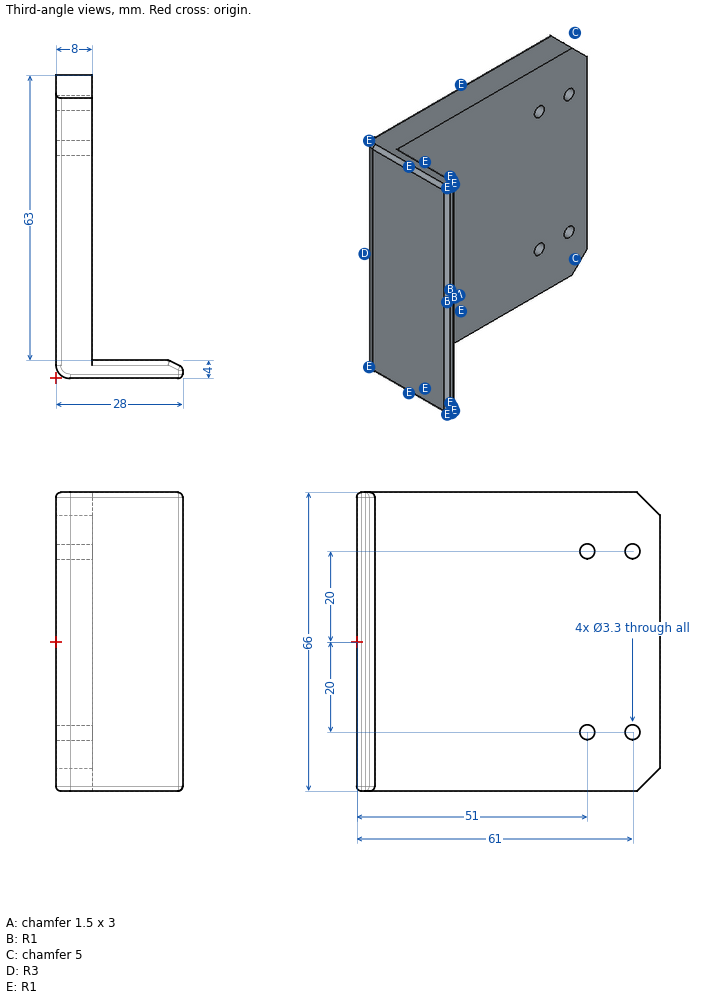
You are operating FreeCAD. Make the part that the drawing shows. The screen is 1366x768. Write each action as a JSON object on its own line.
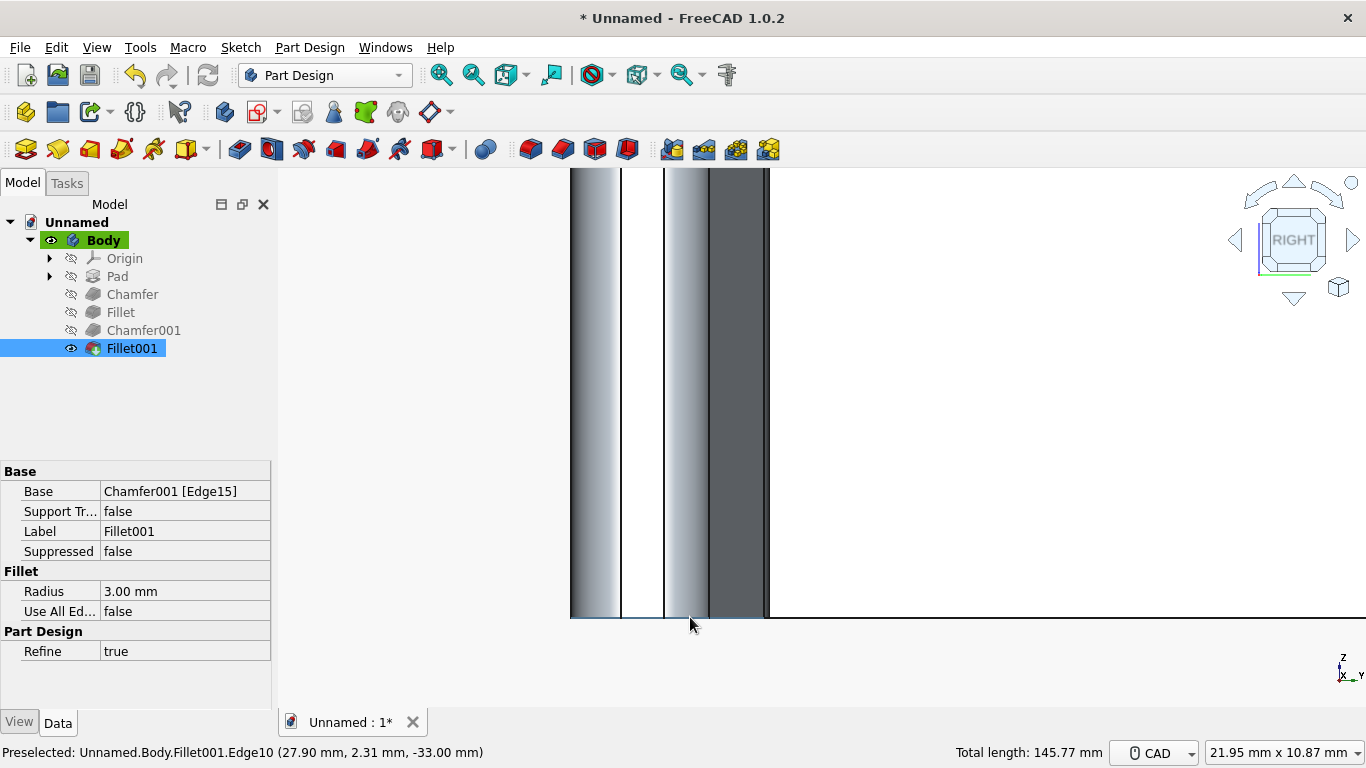
{"action": "left_click", "coordinate": [442, 76]}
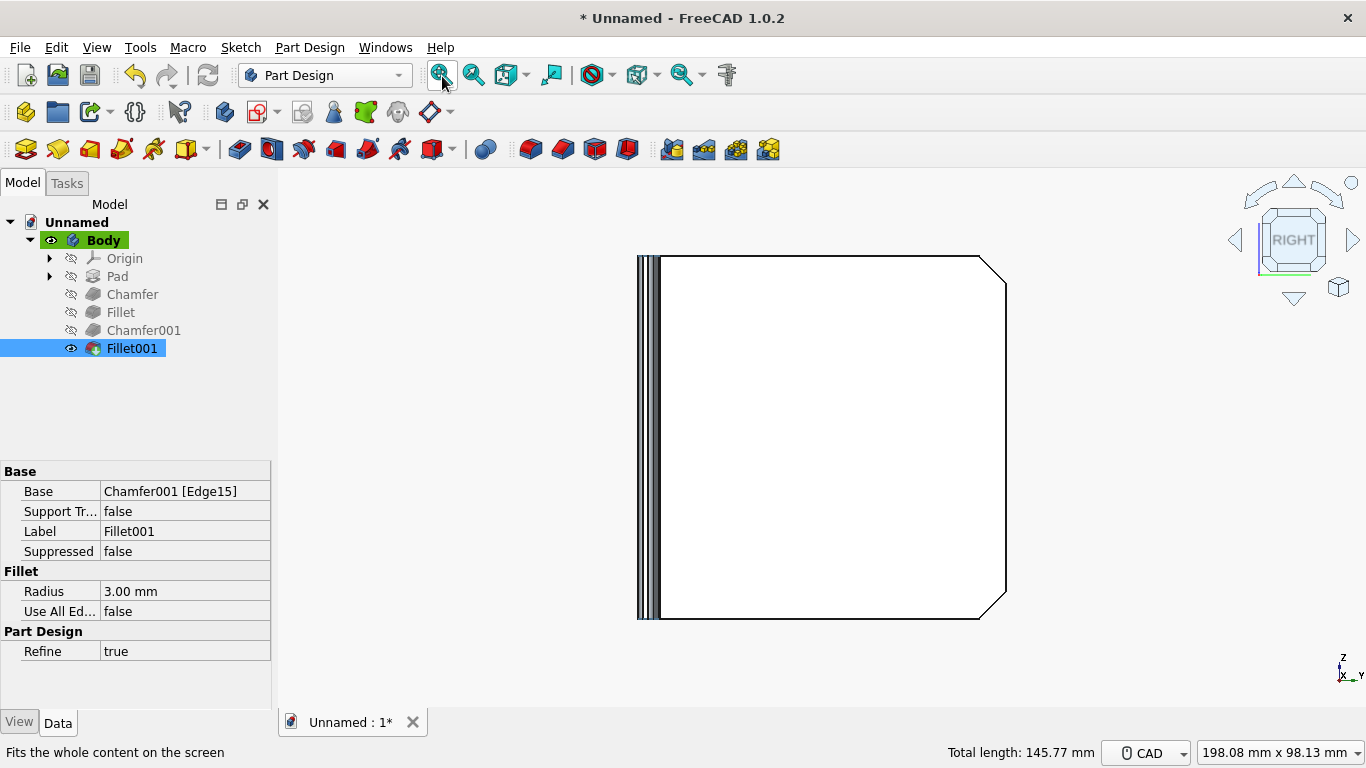
{"action": "key", "text": "5"}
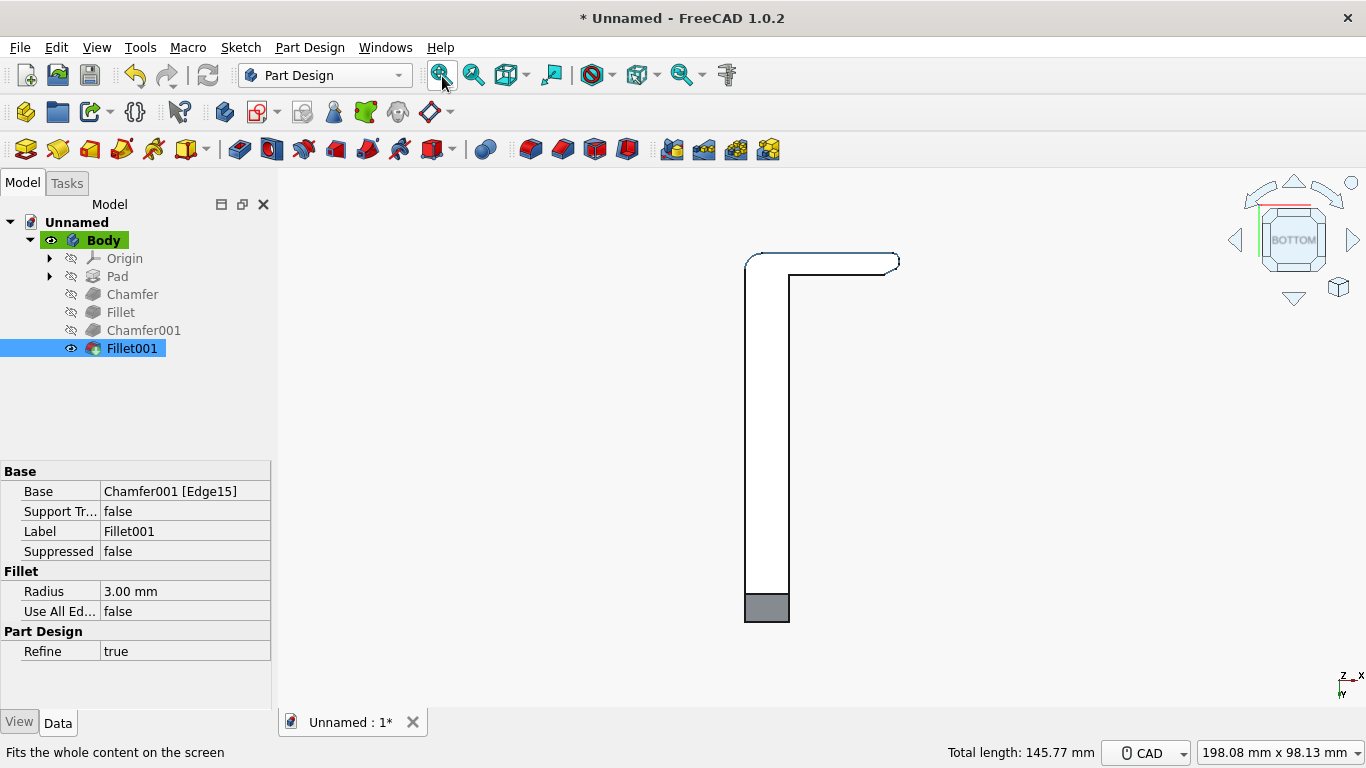
{"action": "left_click", "coordinate": [835, 274], "text": "ctrl"}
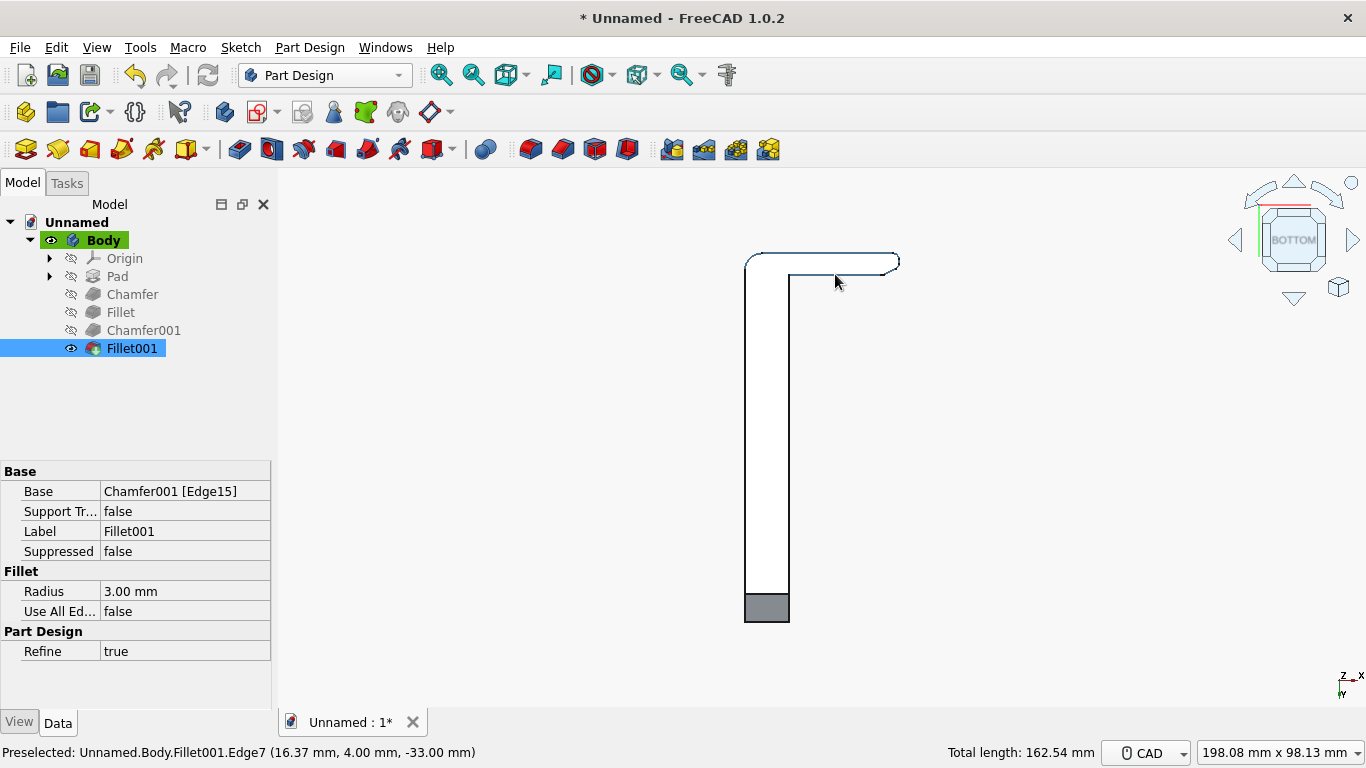
{"action": "left_click", "coordinate": [745, 431], "text": "ctrl"}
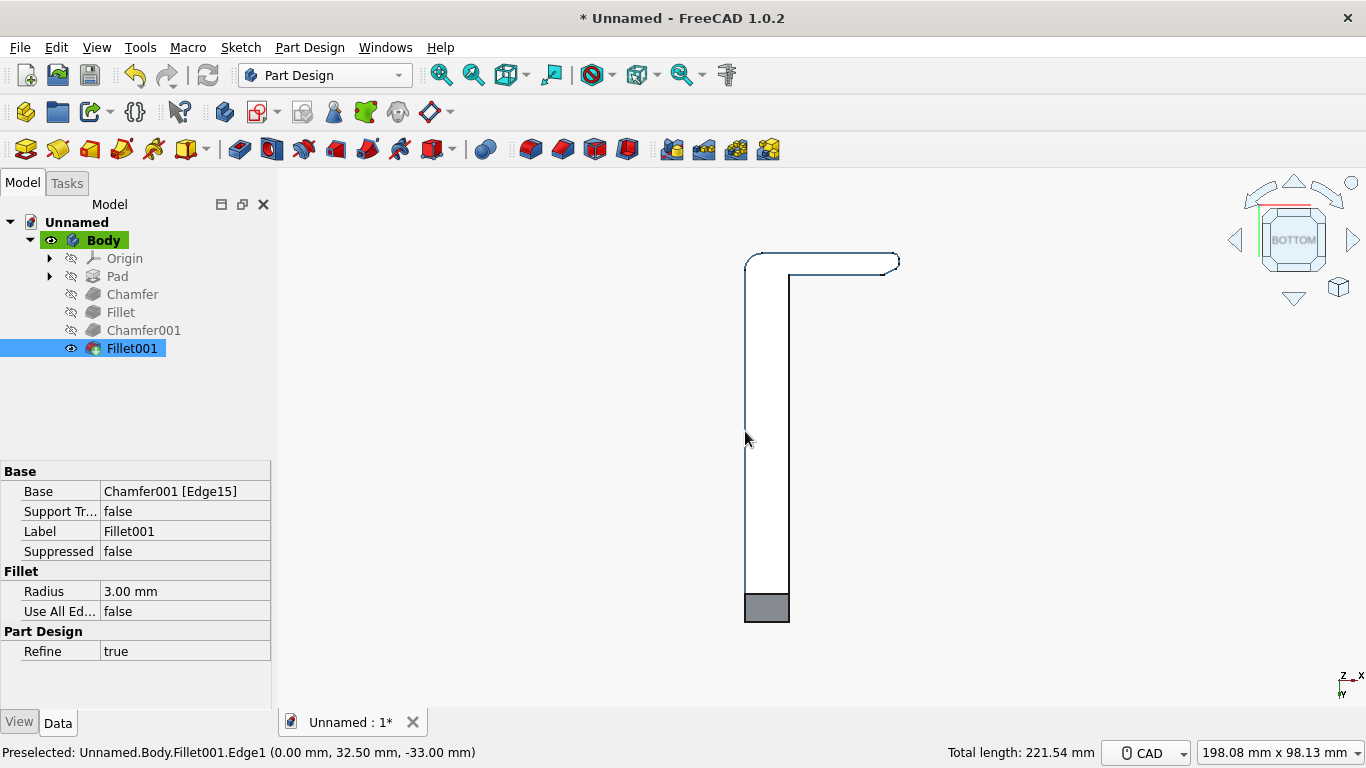
{"action": "scroll", "coordinate": [882, 274], "scroll_direction": "up", "scroll_amount": 14}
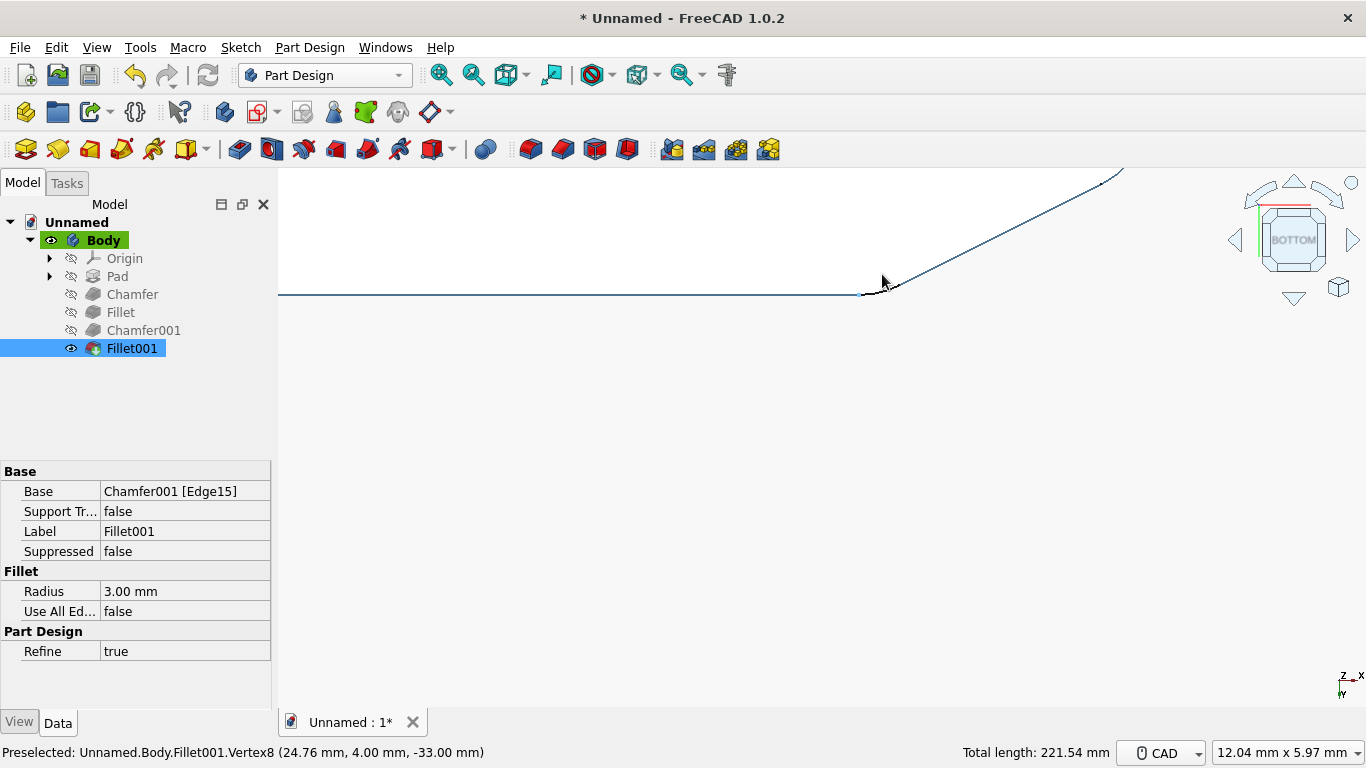
{"action": "left_click", "coordinate": [880, 292], "text": "ctrl"}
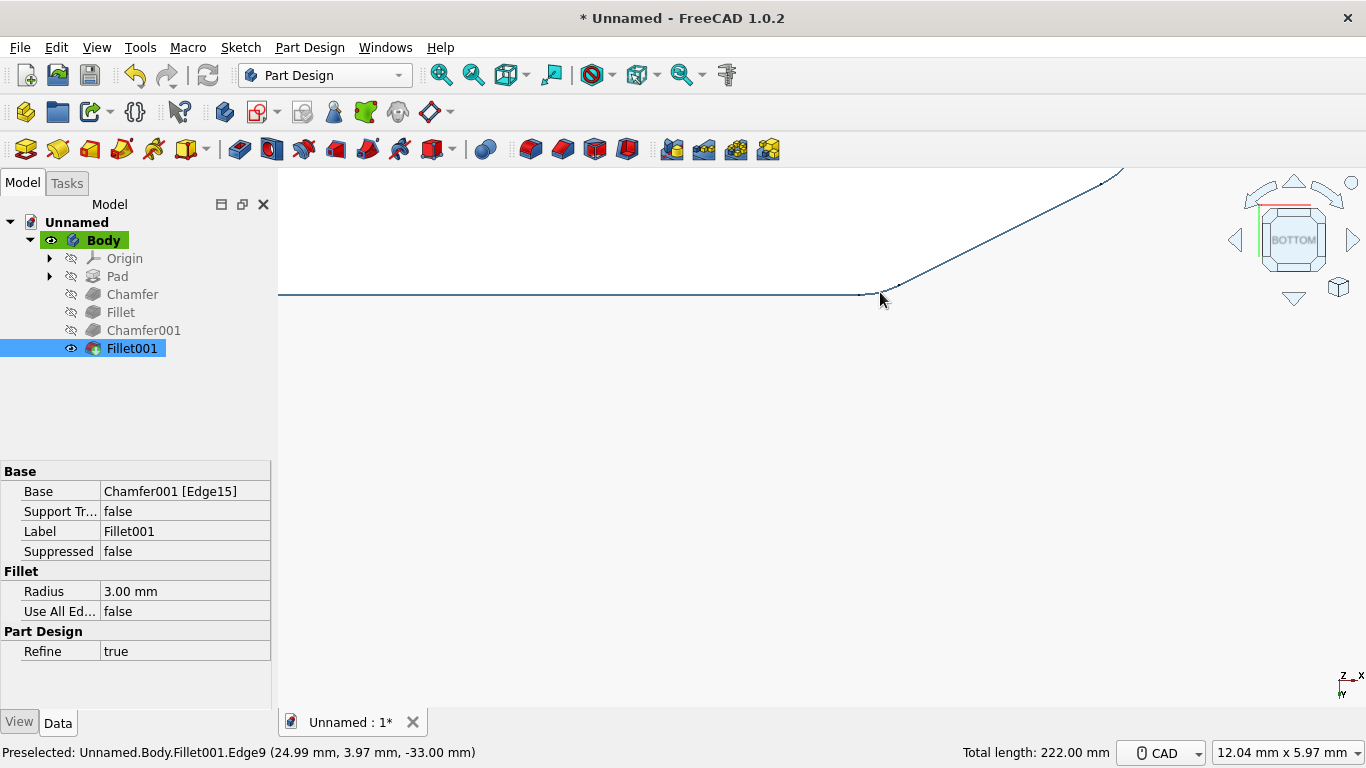
{"action": "left_click", "coordinate": [532, 150]}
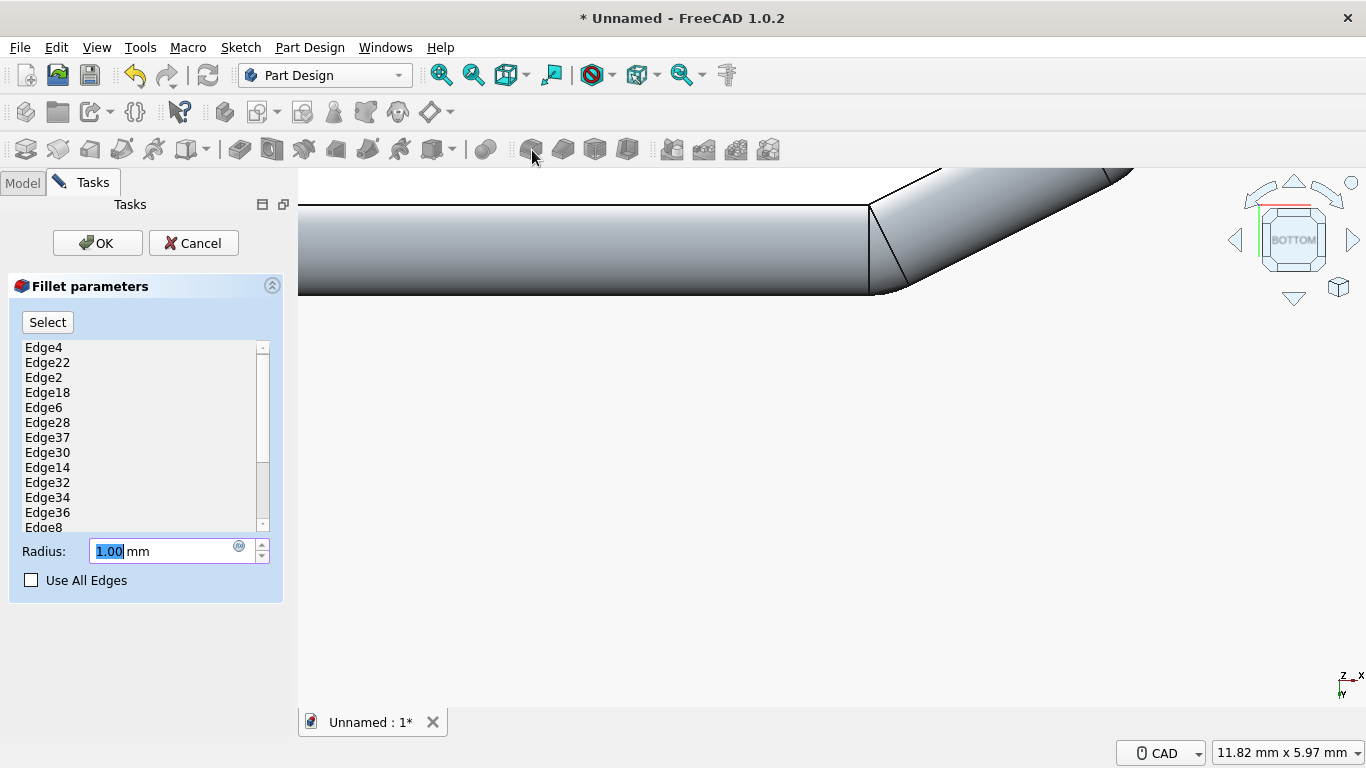
{"action": "type", "text": "1"}
{"action": "key", "text": "Tab"}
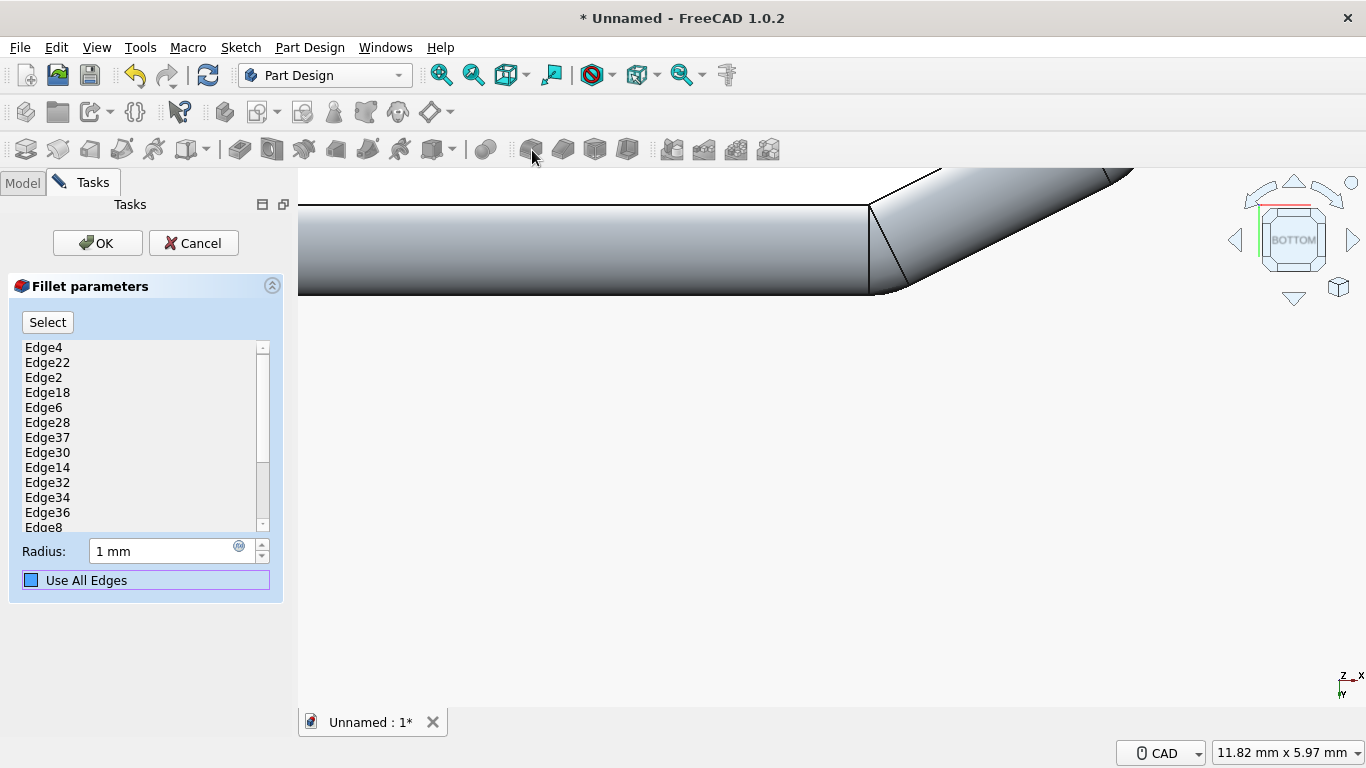
{"action": "left_click", "coordinate": [98, 243]}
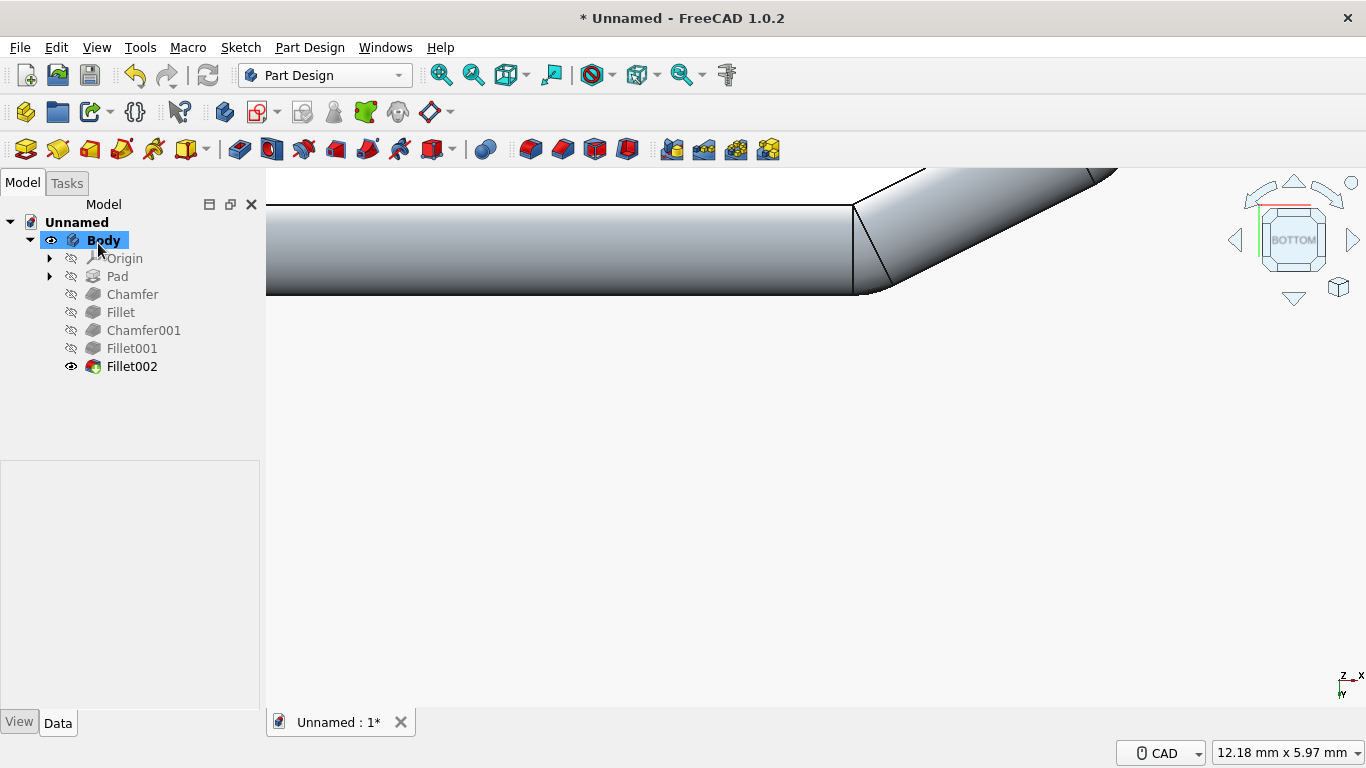
{"action": "left_click", "coordinate": [442, 76]}